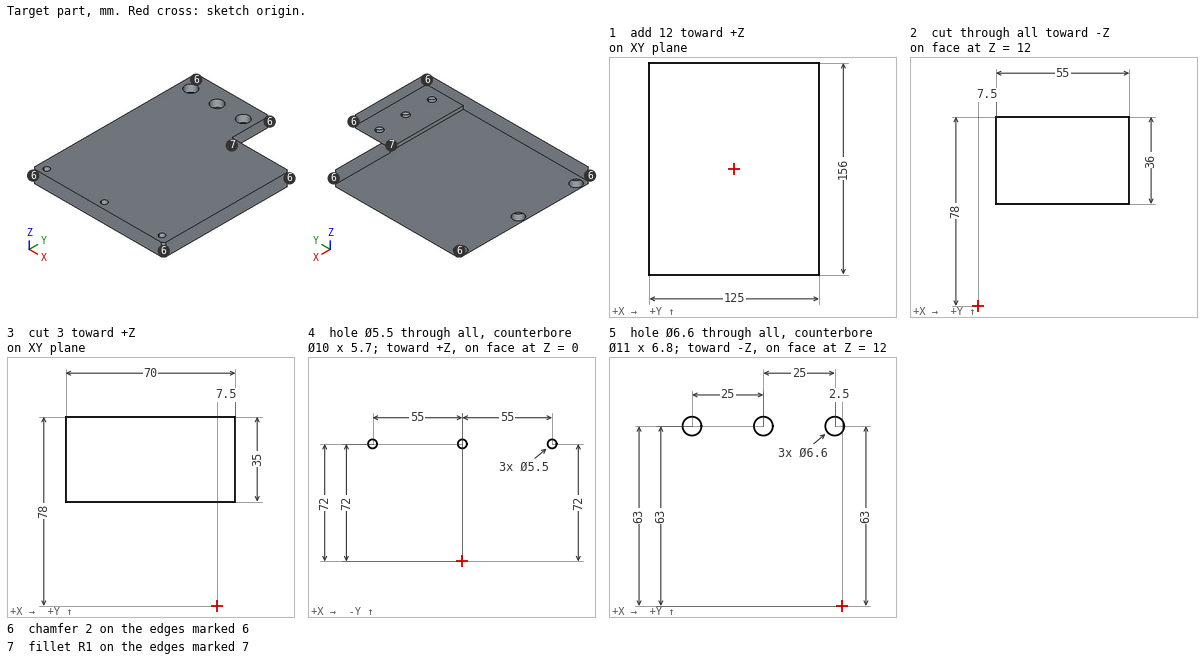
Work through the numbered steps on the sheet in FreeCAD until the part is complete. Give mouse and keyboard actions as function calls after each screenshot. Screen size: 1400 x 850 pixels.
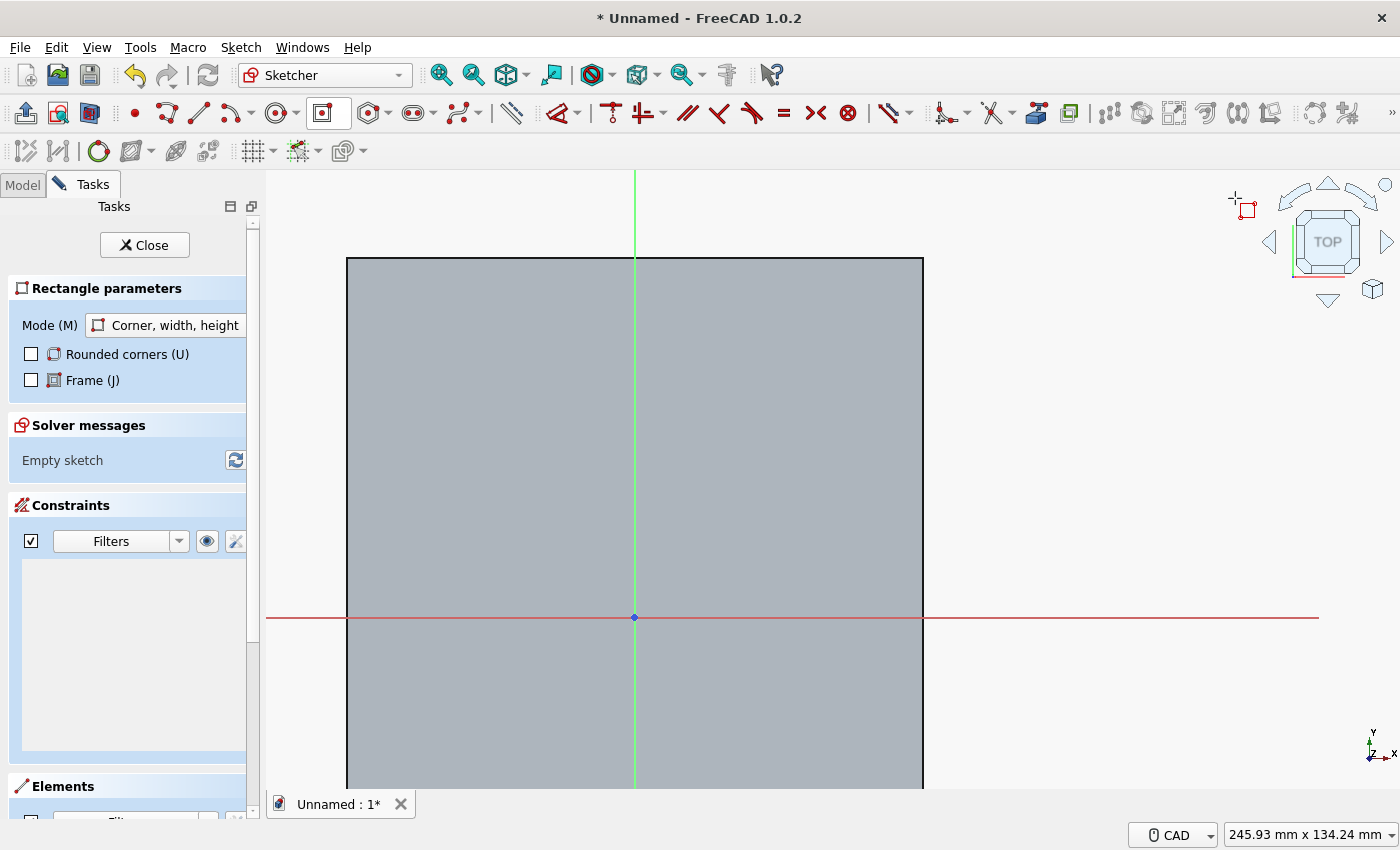
click(669, 258)
move(923, 424)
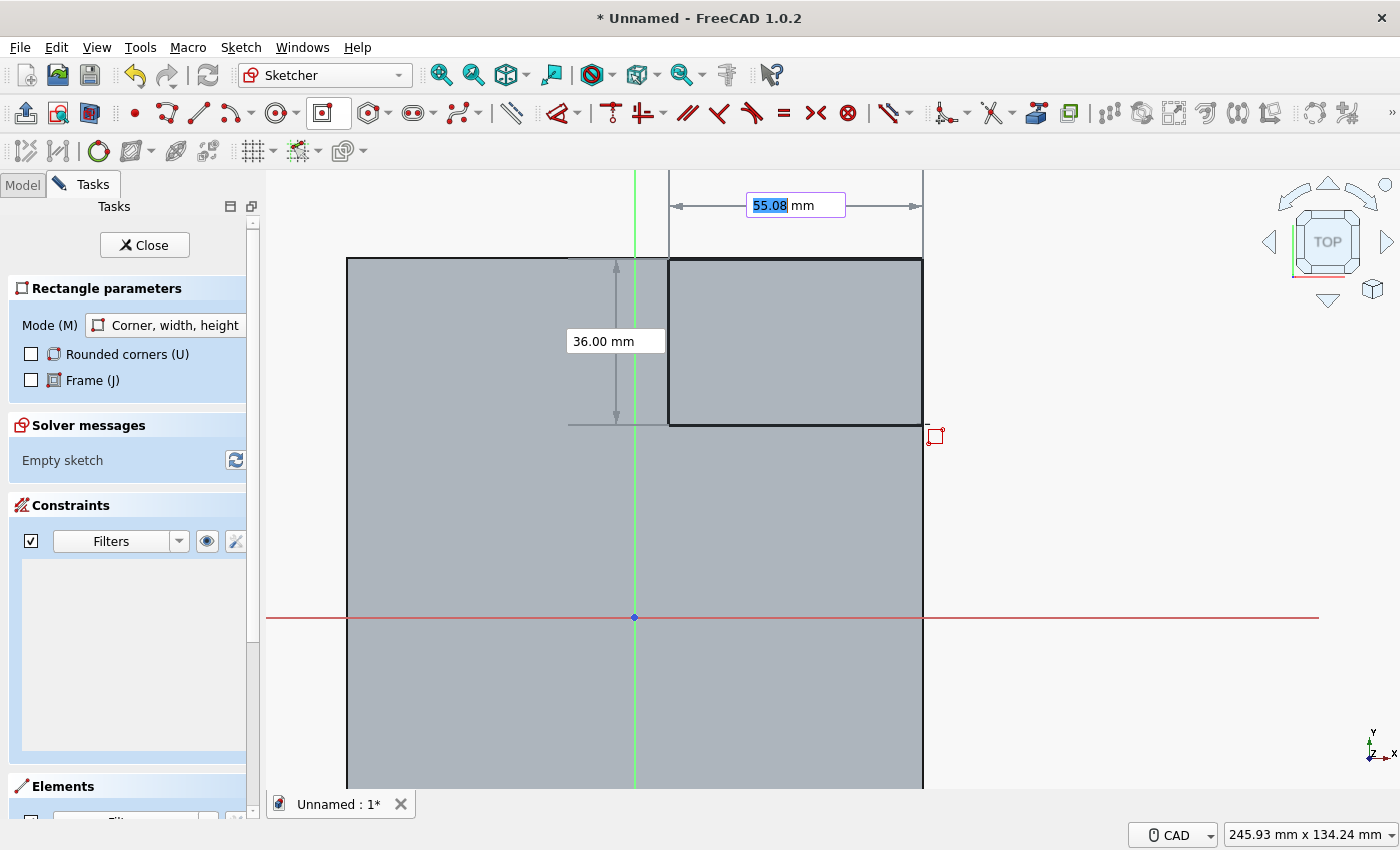
text(55)
key(Tab)
text(36)
key(Return)
key(Escape)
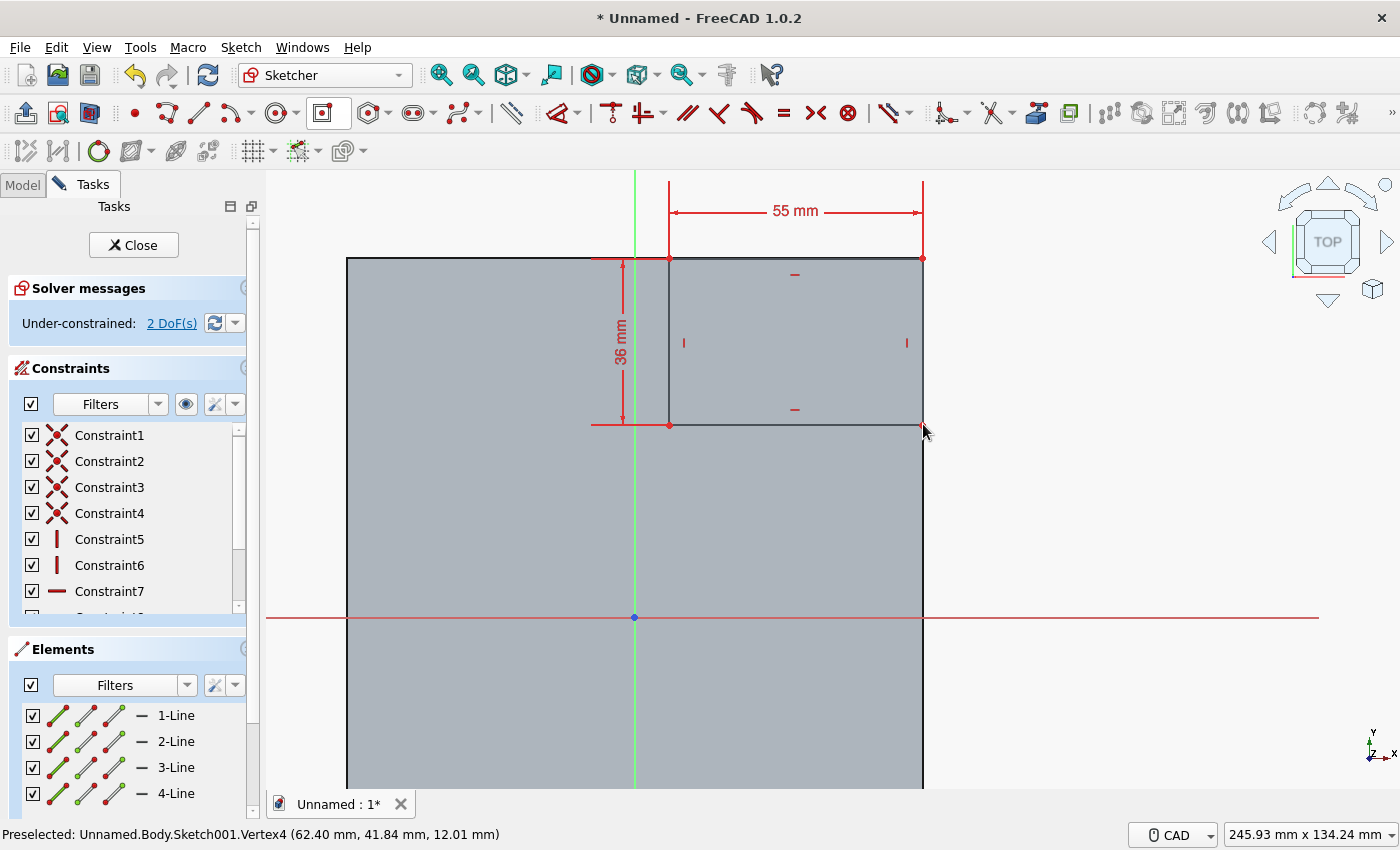
click(558, 114)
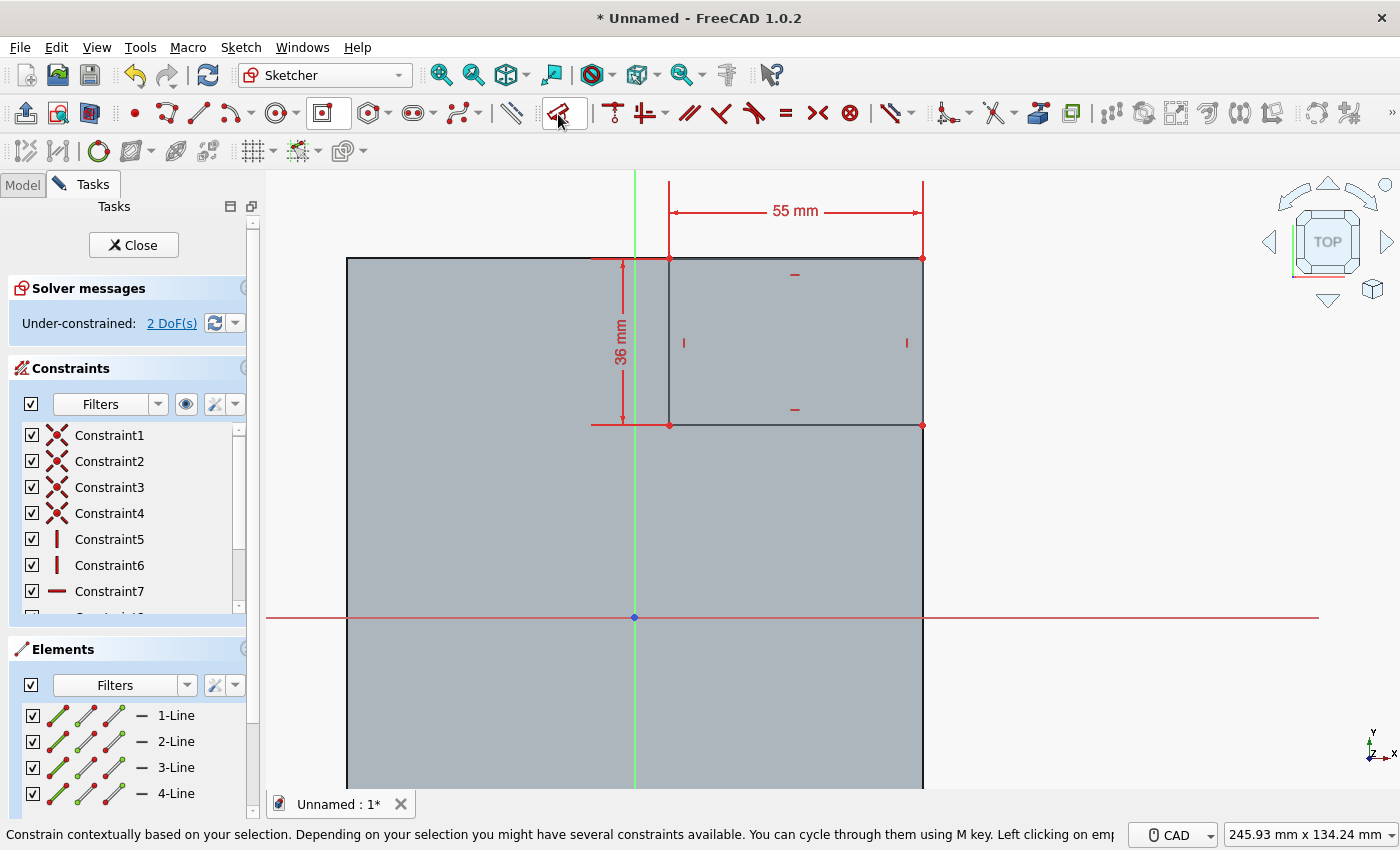
click(669, 259)
click(601, 438)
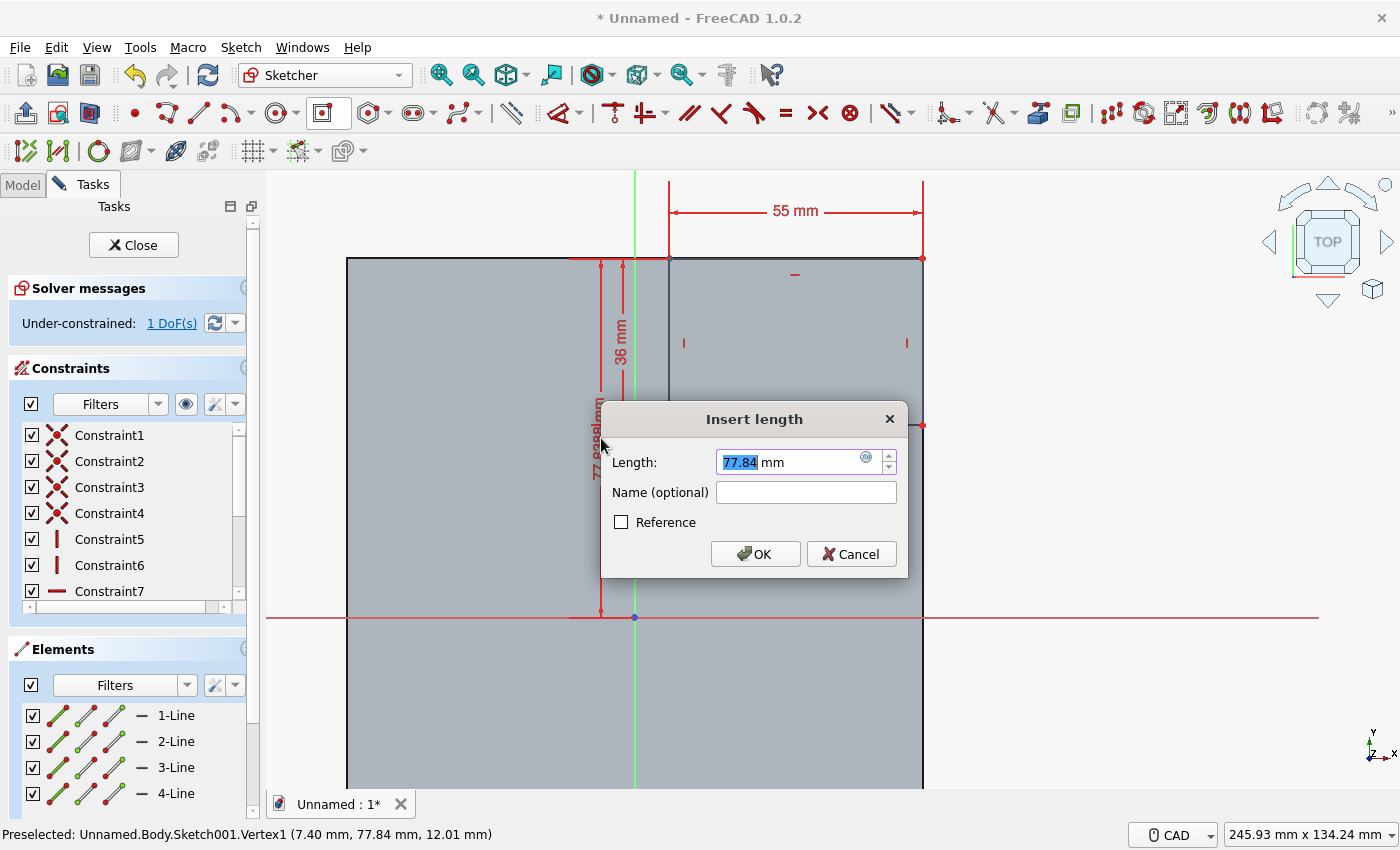
text(78)
key(Return)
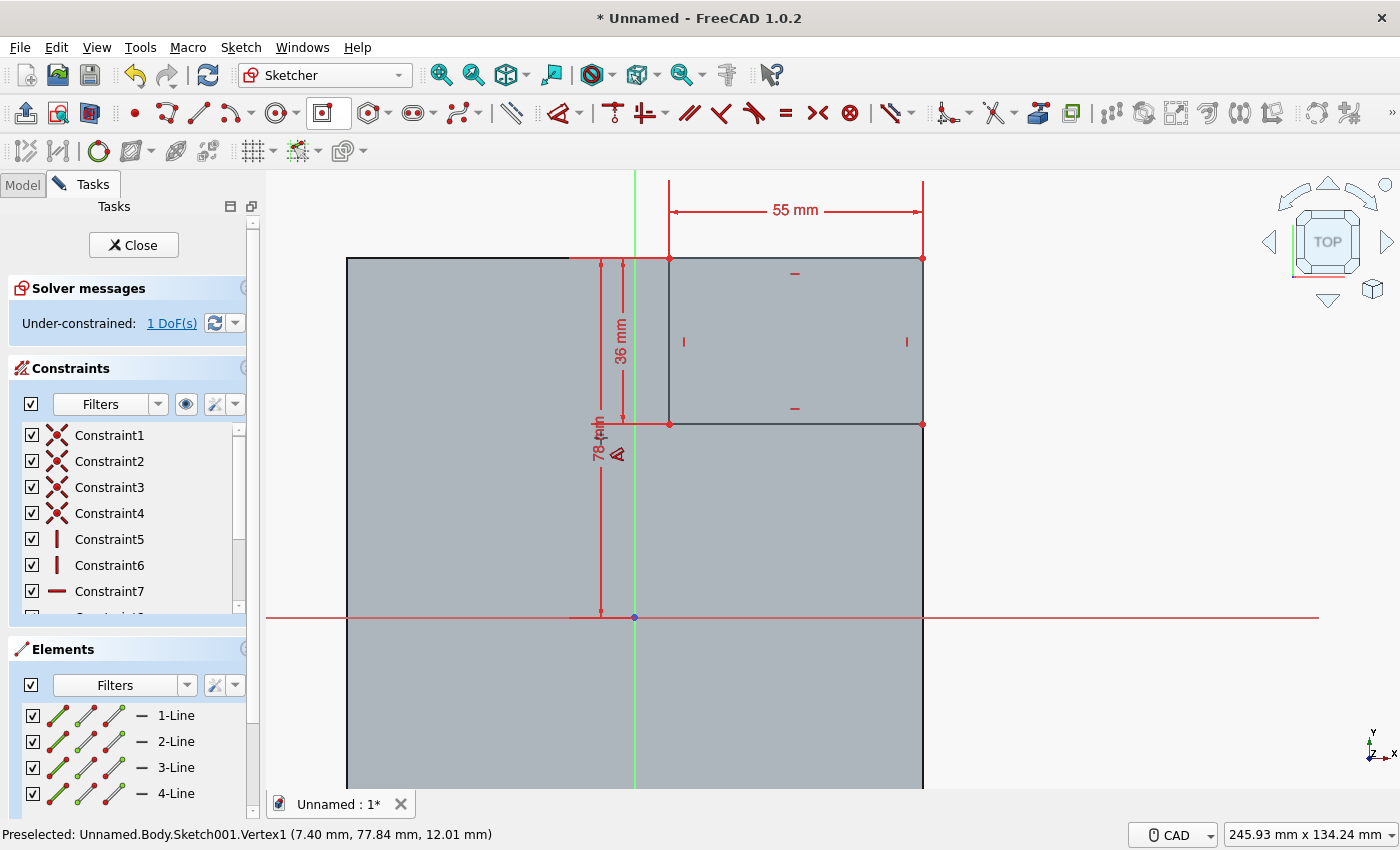
click(669, 258)
click(652, 652)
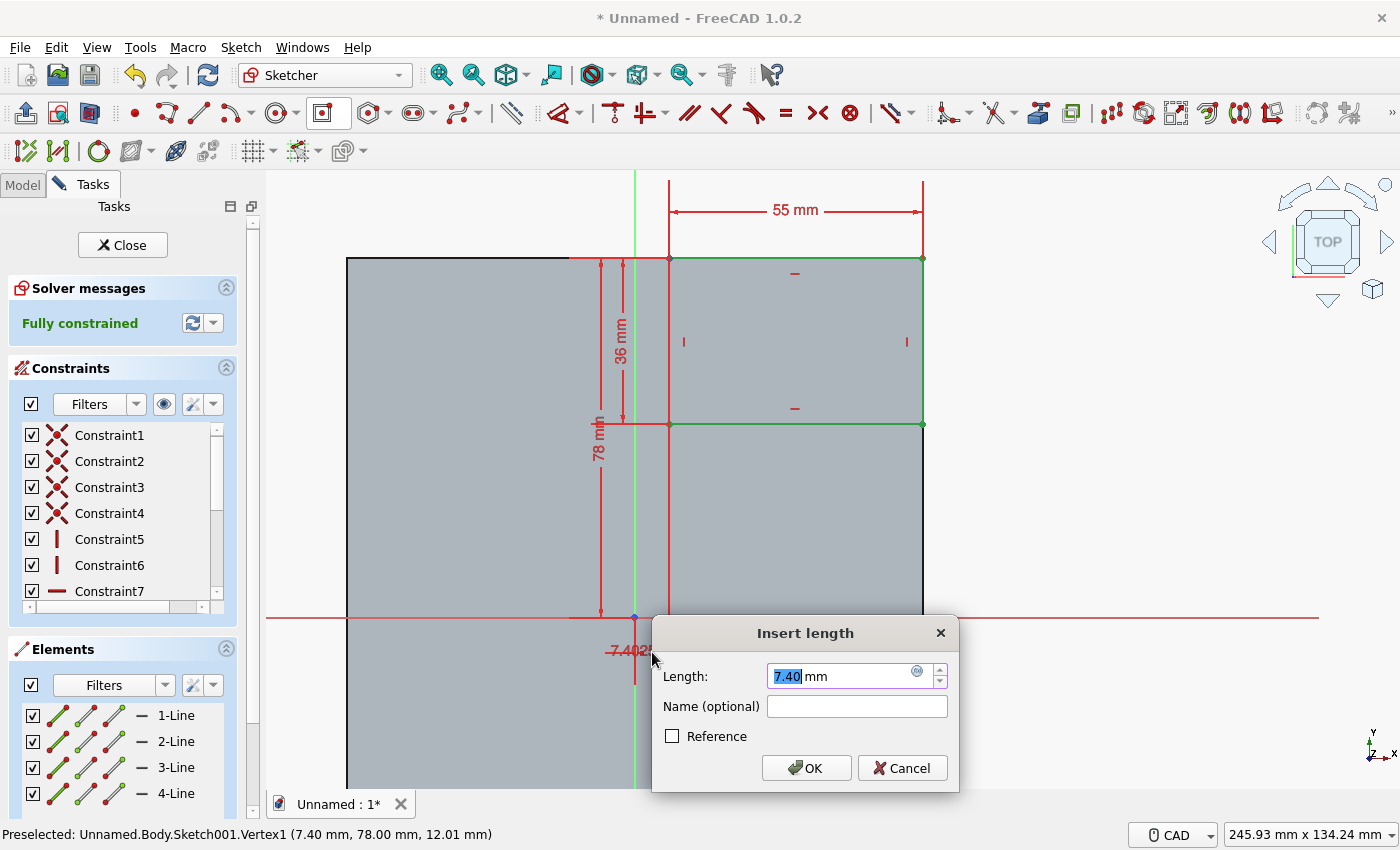
text(7.5)
key(Return)
key(Escape)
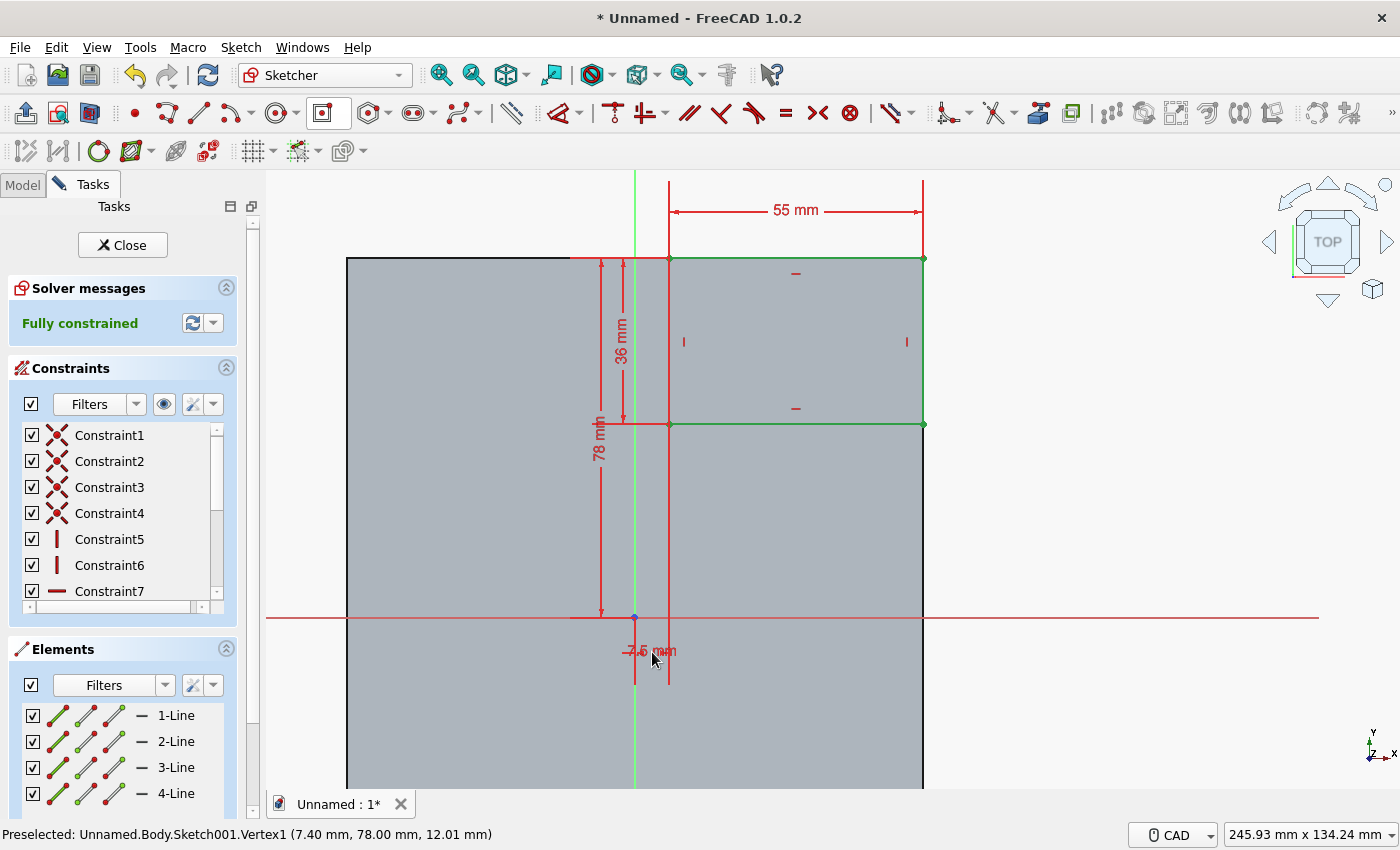
click(123, 245)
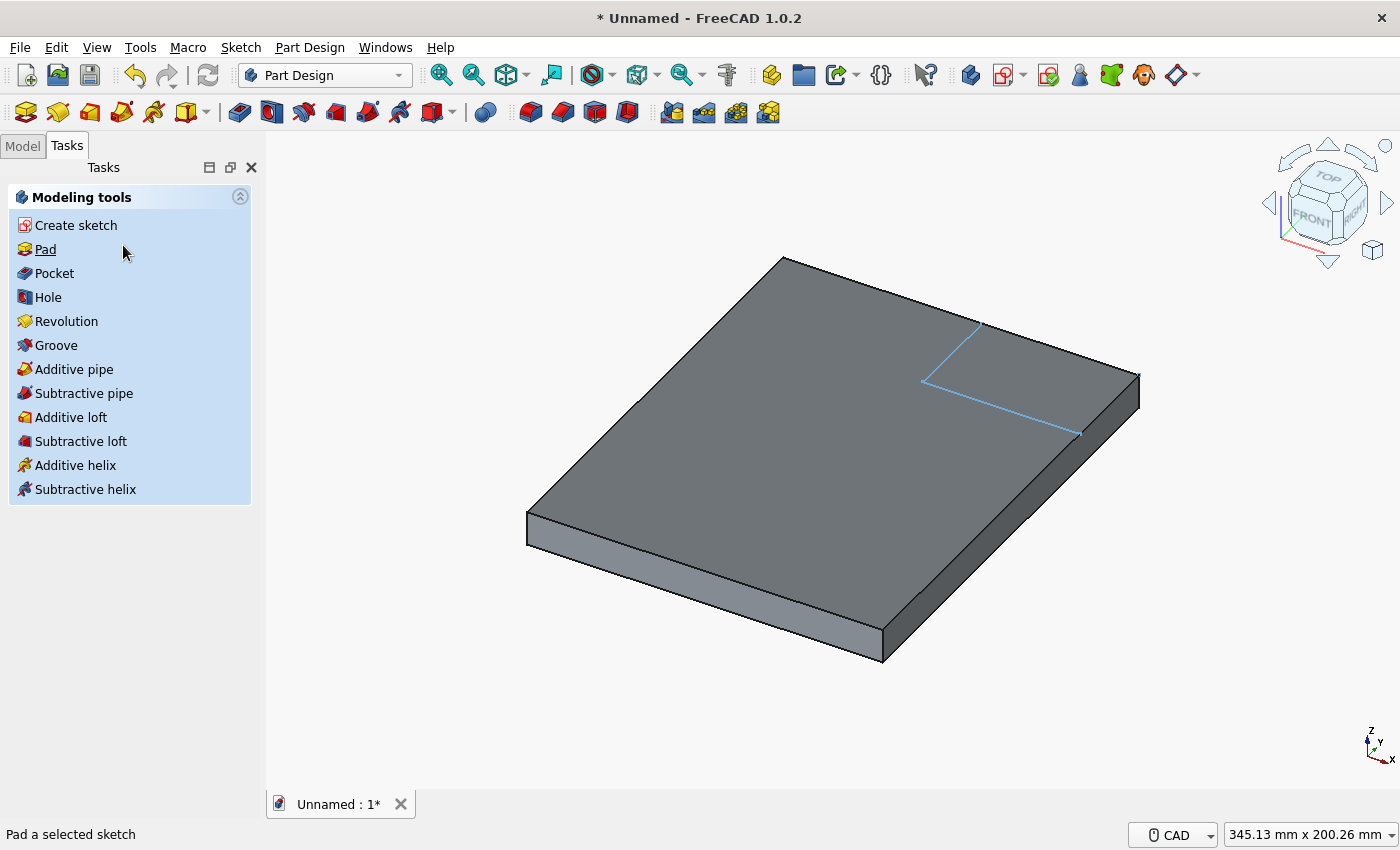
click(240, 112)